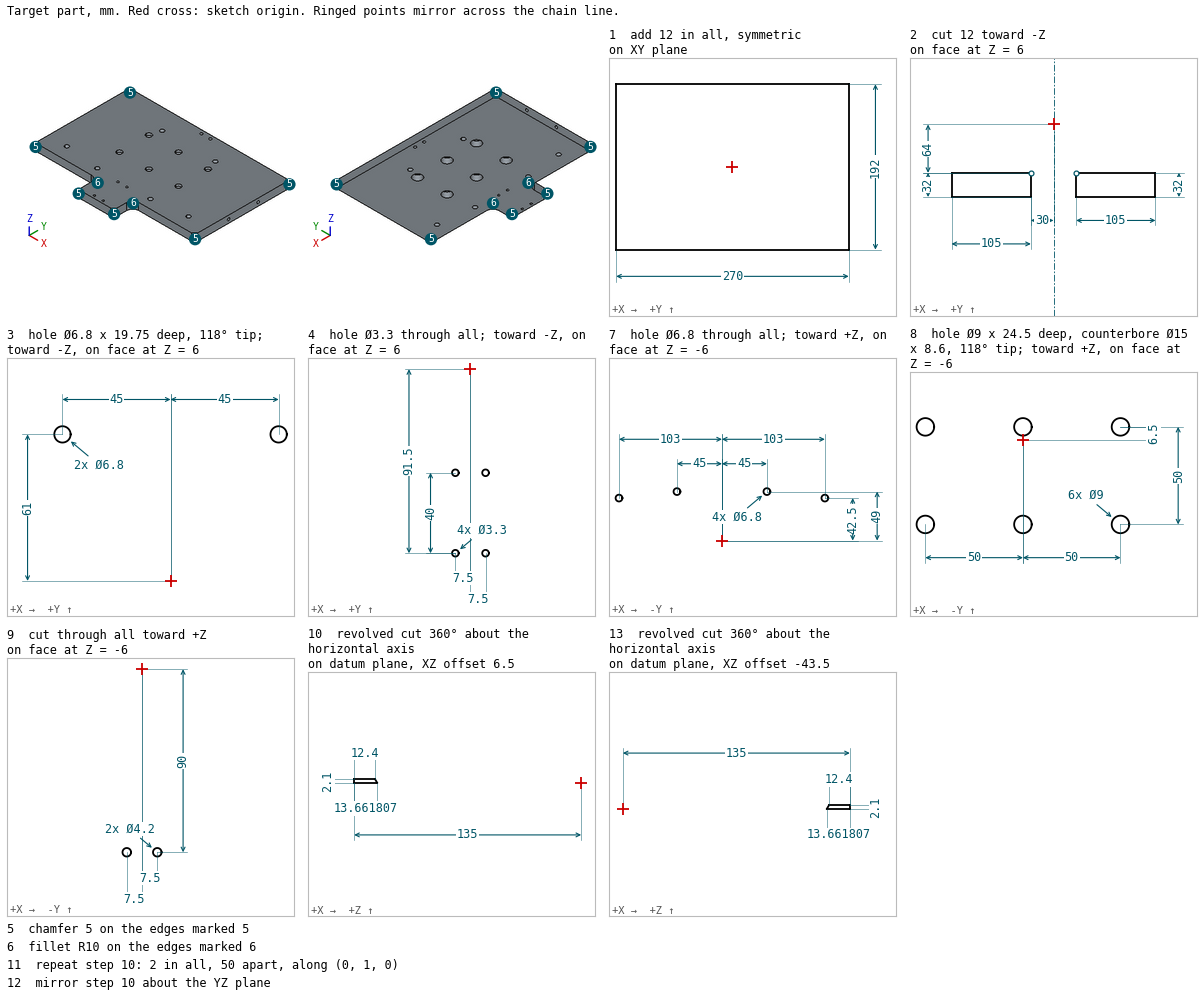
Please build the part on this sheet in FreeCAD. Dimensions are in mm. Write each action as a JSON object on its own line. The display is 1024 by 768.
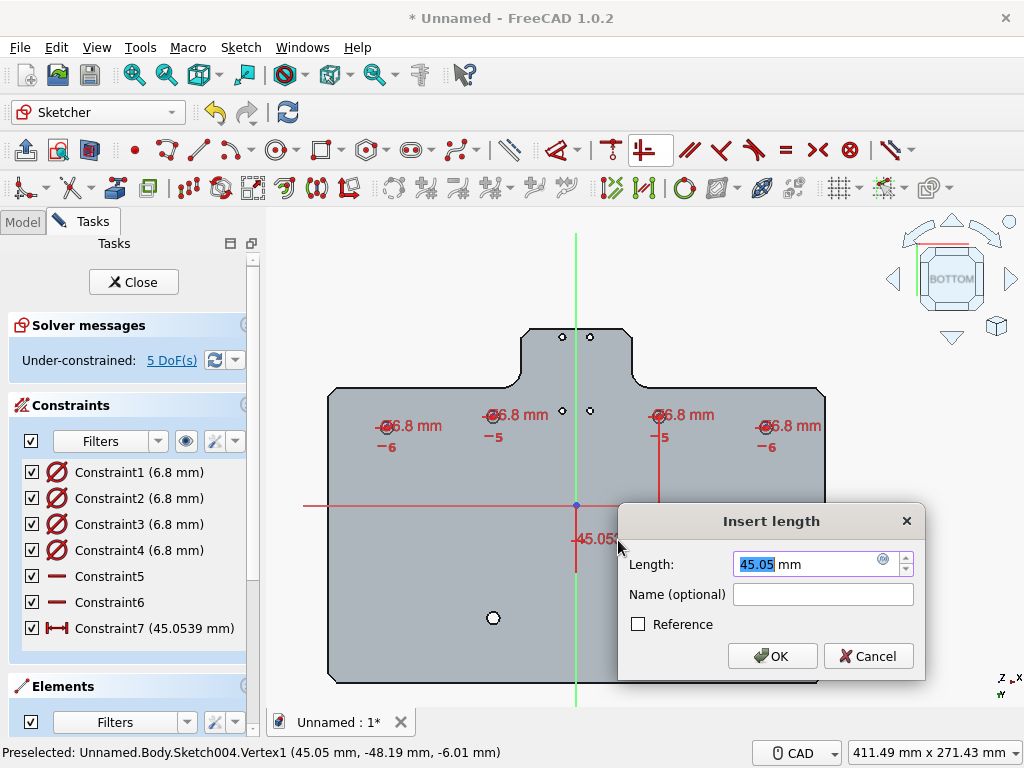
{"action": "type", "text": "45"}
{"action": "key", "text": "Return"}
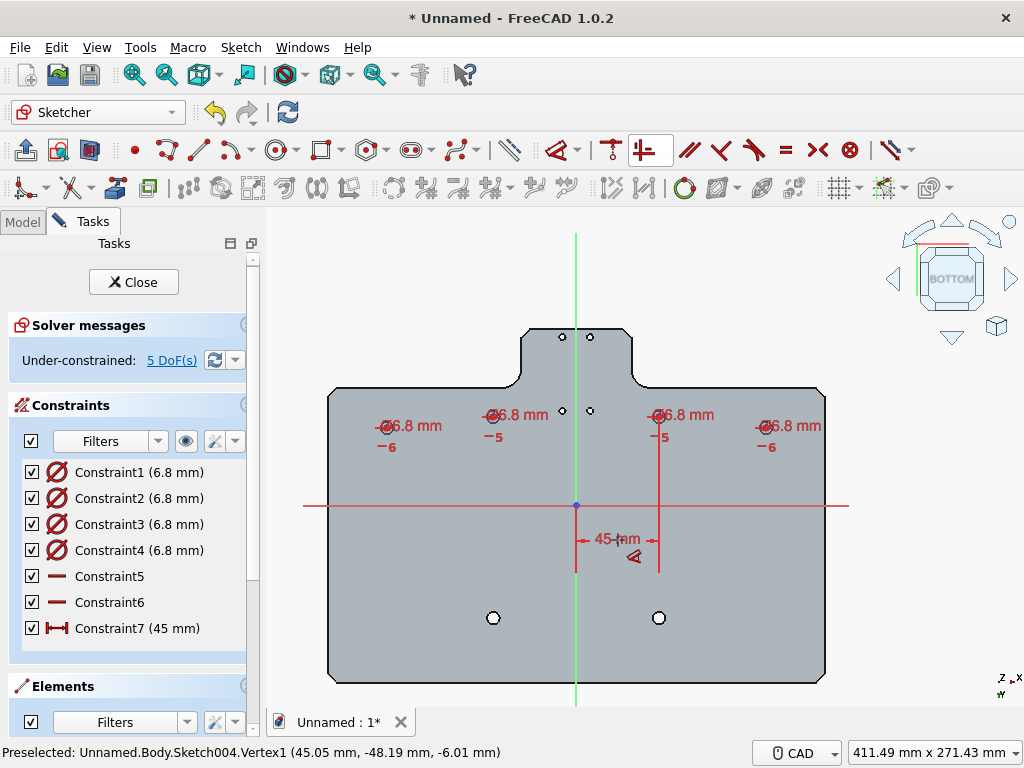
{"action": "left_click", "coordinate": [659, 417]}
{"action": "left_click", "coordinate": [693, 461]}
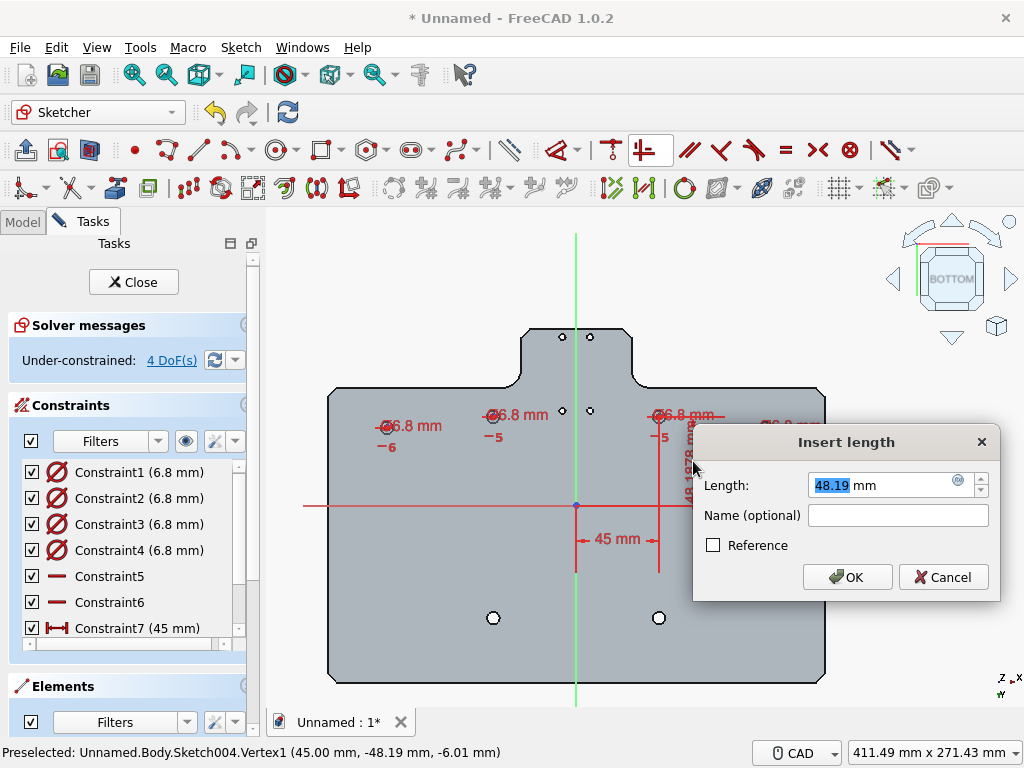
{"action": "type", "text": "49"}
{"action": "key", "text": "Return"}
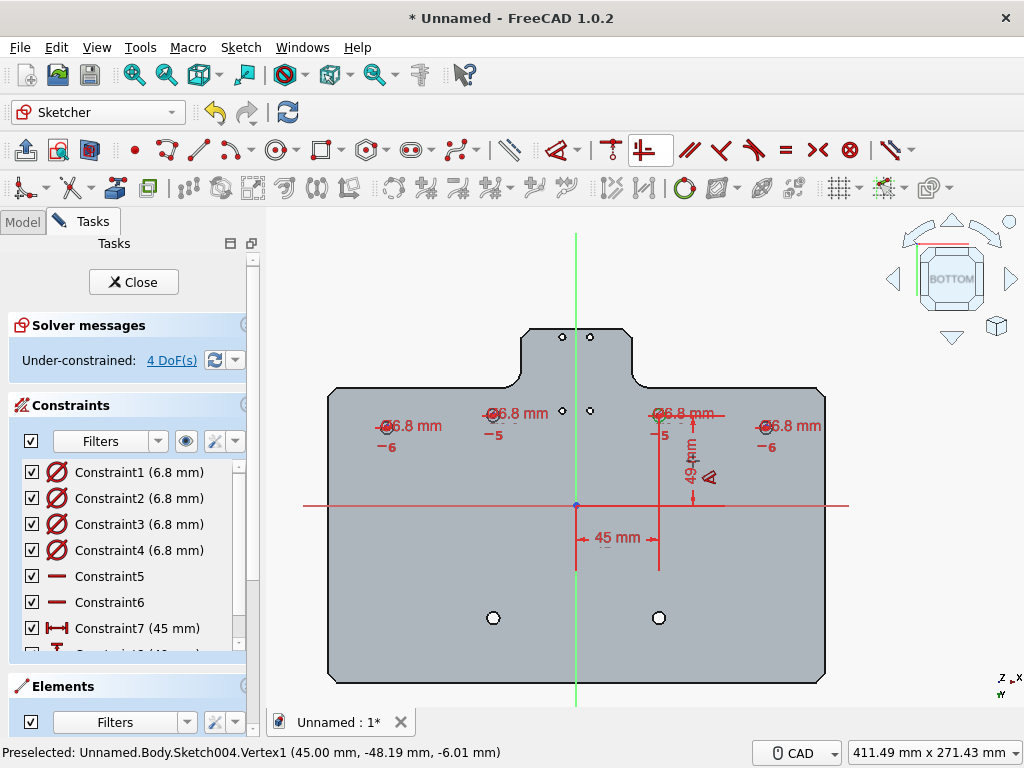
{"action": "left_click", "coordinate": [493, 416]}
{"action": "left_click", "coordinate": [535, 540]}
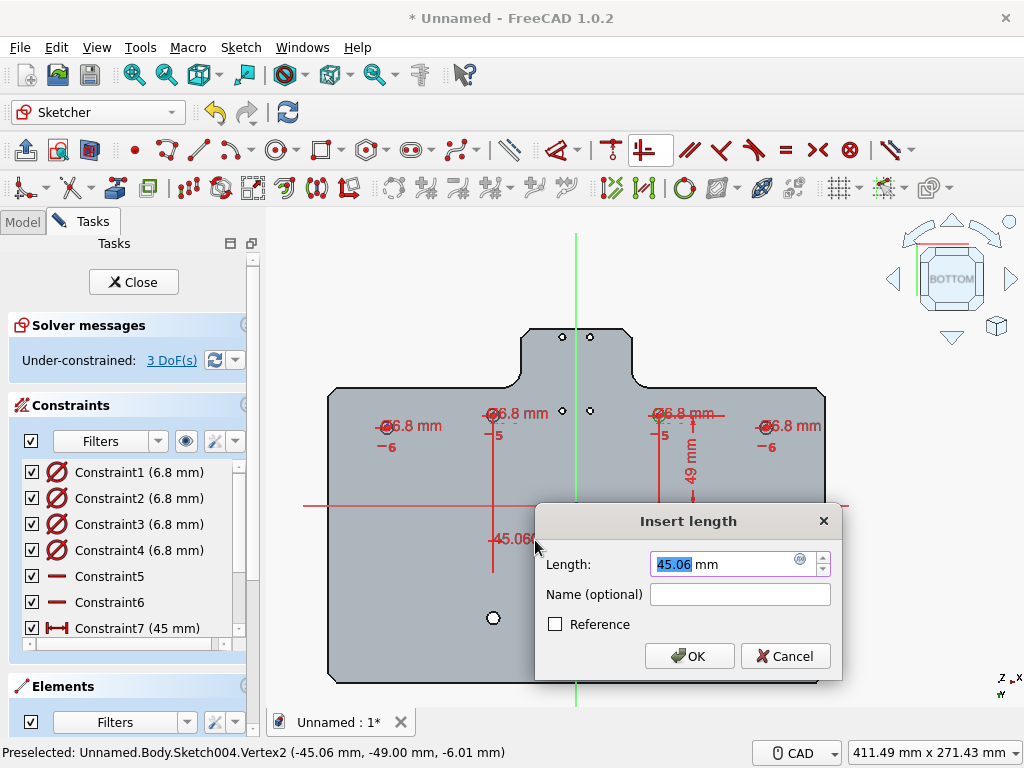
{"action": "type", "text": "45"}
{"action": "key", "text": "Return"}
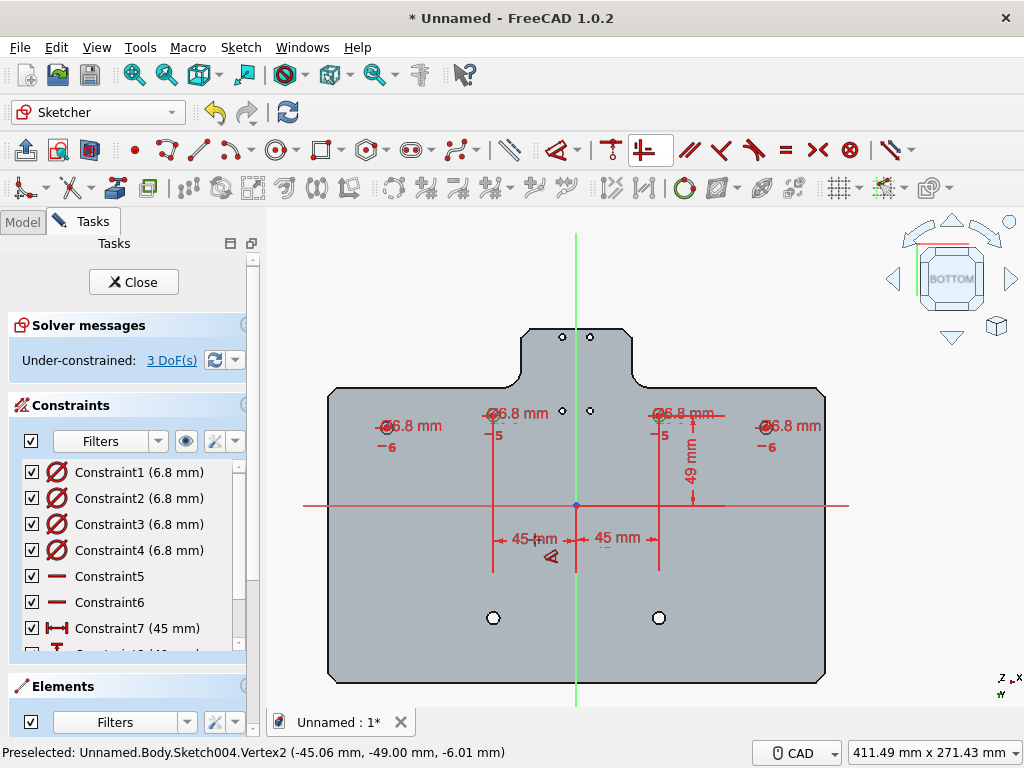
{"action": "left_click", "coordinate": [766, 428]}
{"action": "left_click", "coordinate": [715, 540]}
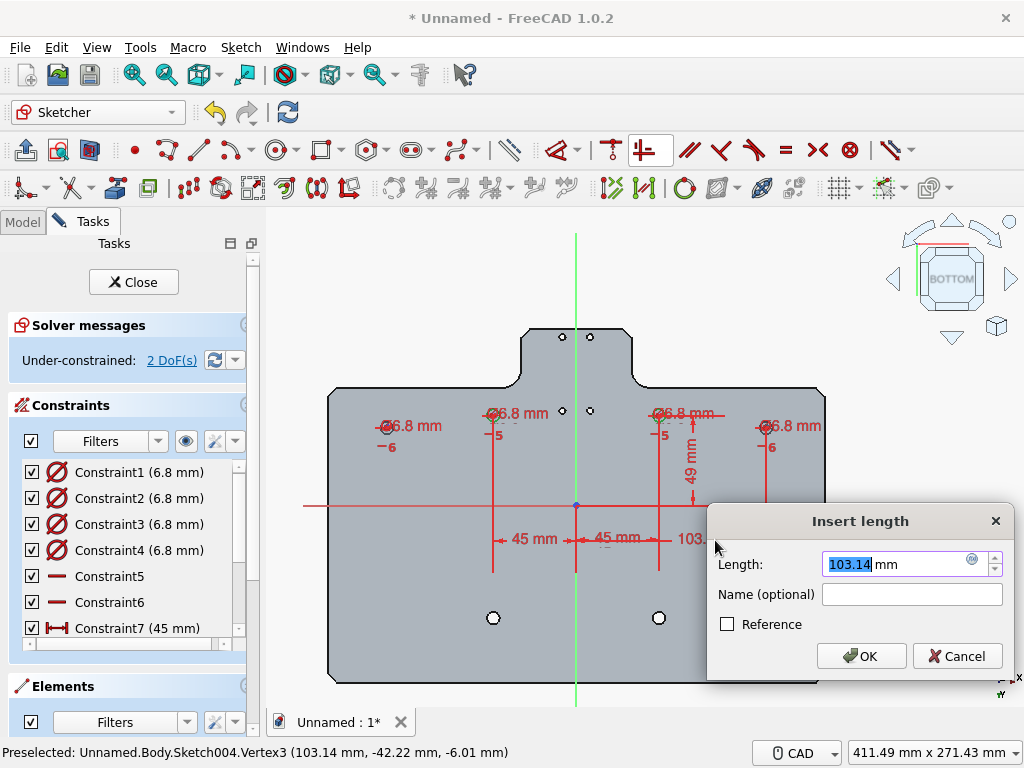
{"action": "type", "text": "103"}
{"action": "key", "text": "Return"}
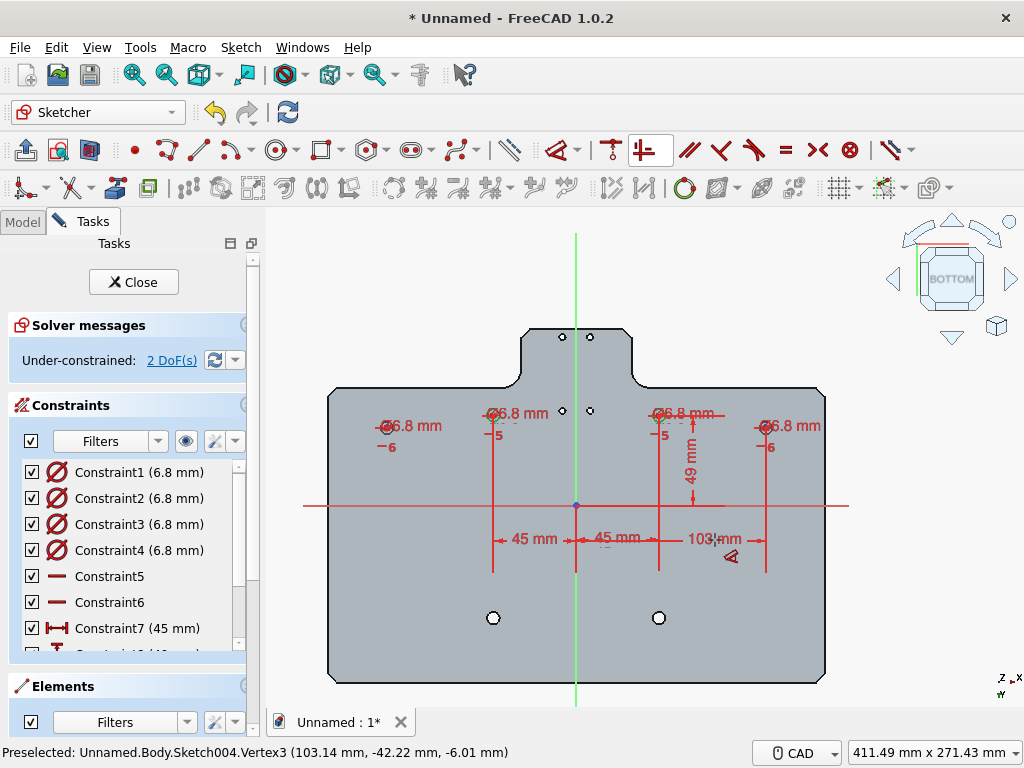
{"action": "left_click", "coordinate": [387, 428]}
{"action": "left_click", "coordinate": [438, 540]}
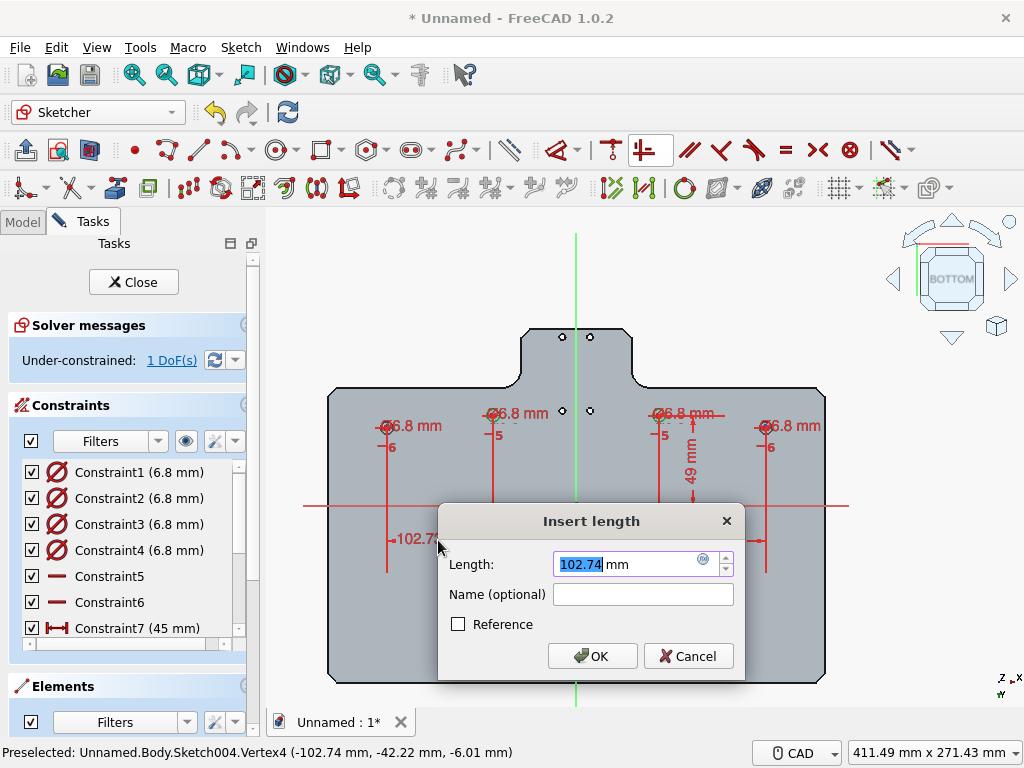
{"action": "type", "text": "103"}
{"action": "key", "text": "Return"}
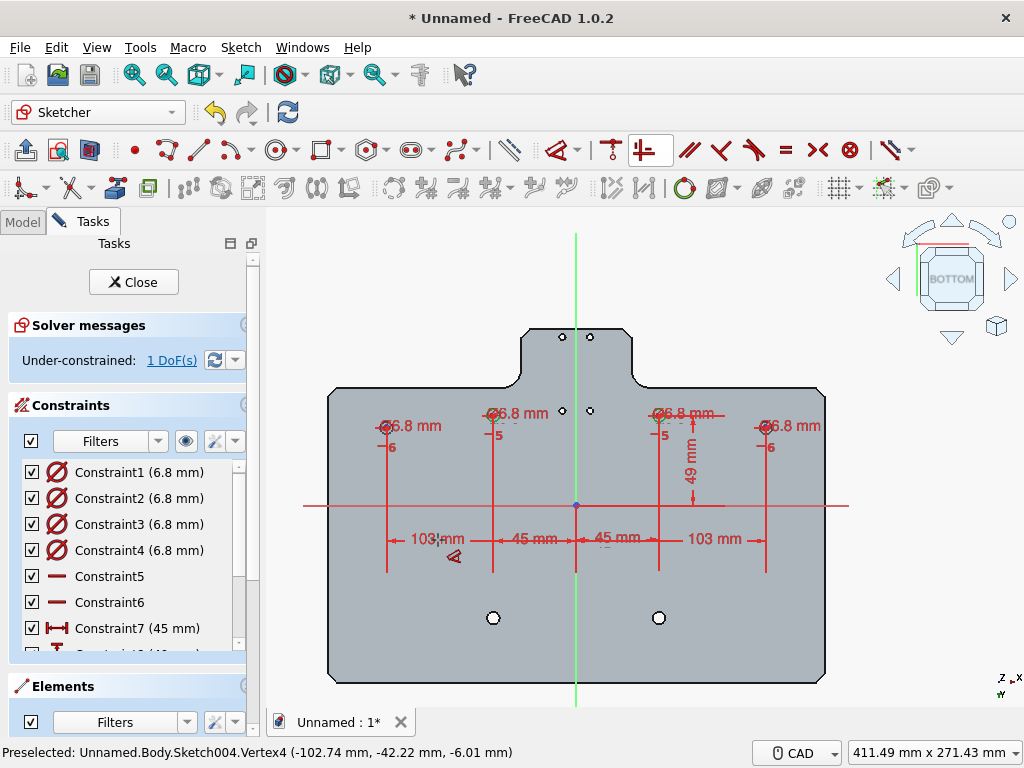
{"action": "left_click", "coordinate": [766, 428]}
{"action": "left_click", "coordinate": [800, 467]}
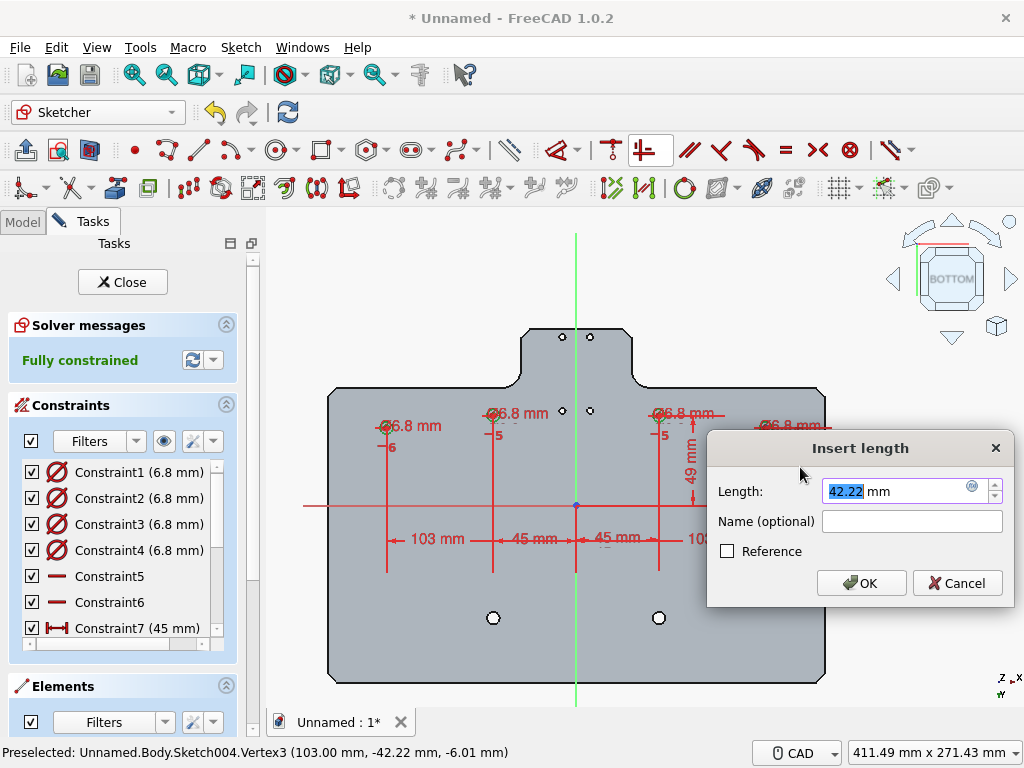
{"action": "type", "text": "42.5"}
{"action": "key", "text": "Return"}
{"action": "key", "text": "Escape"}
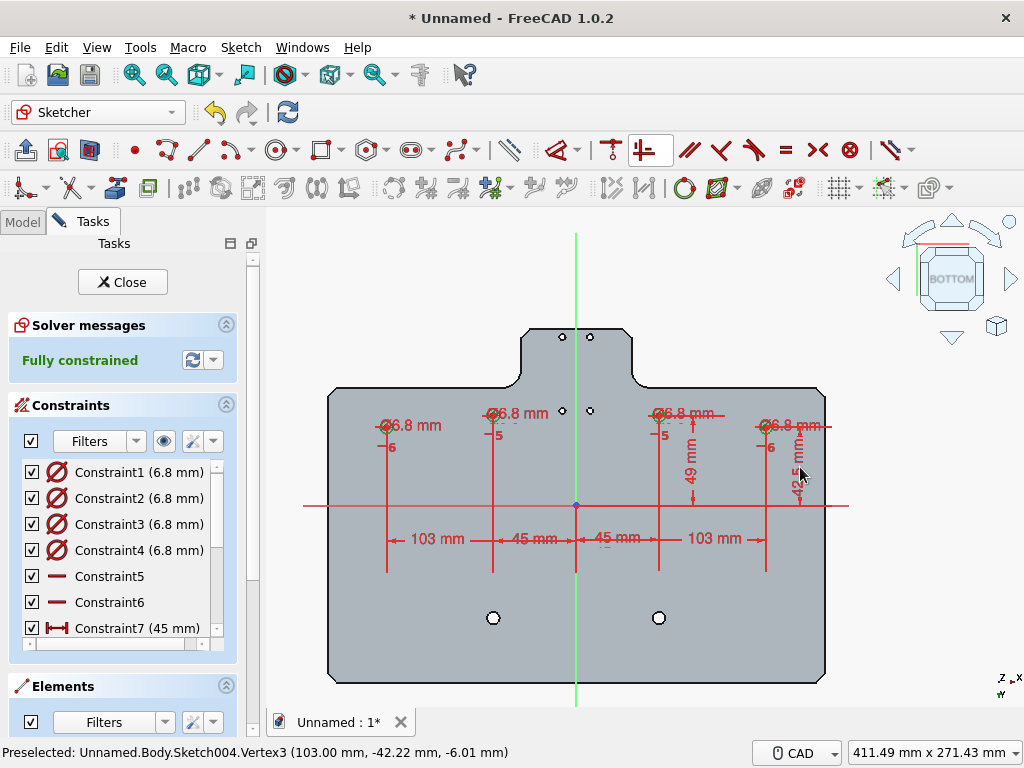
{"action": "left_click", "coordinate": [123, 282]}